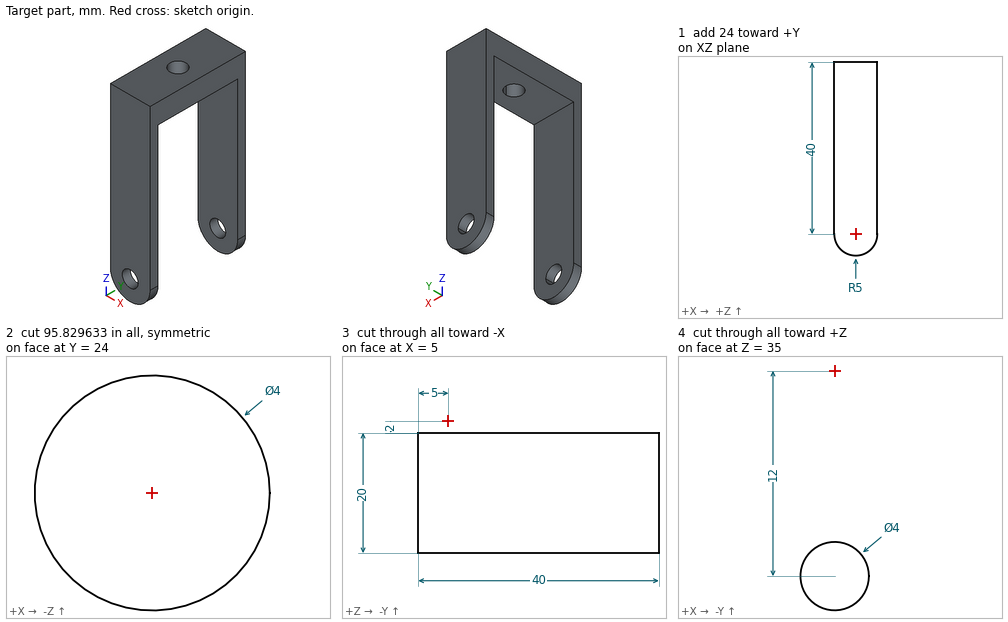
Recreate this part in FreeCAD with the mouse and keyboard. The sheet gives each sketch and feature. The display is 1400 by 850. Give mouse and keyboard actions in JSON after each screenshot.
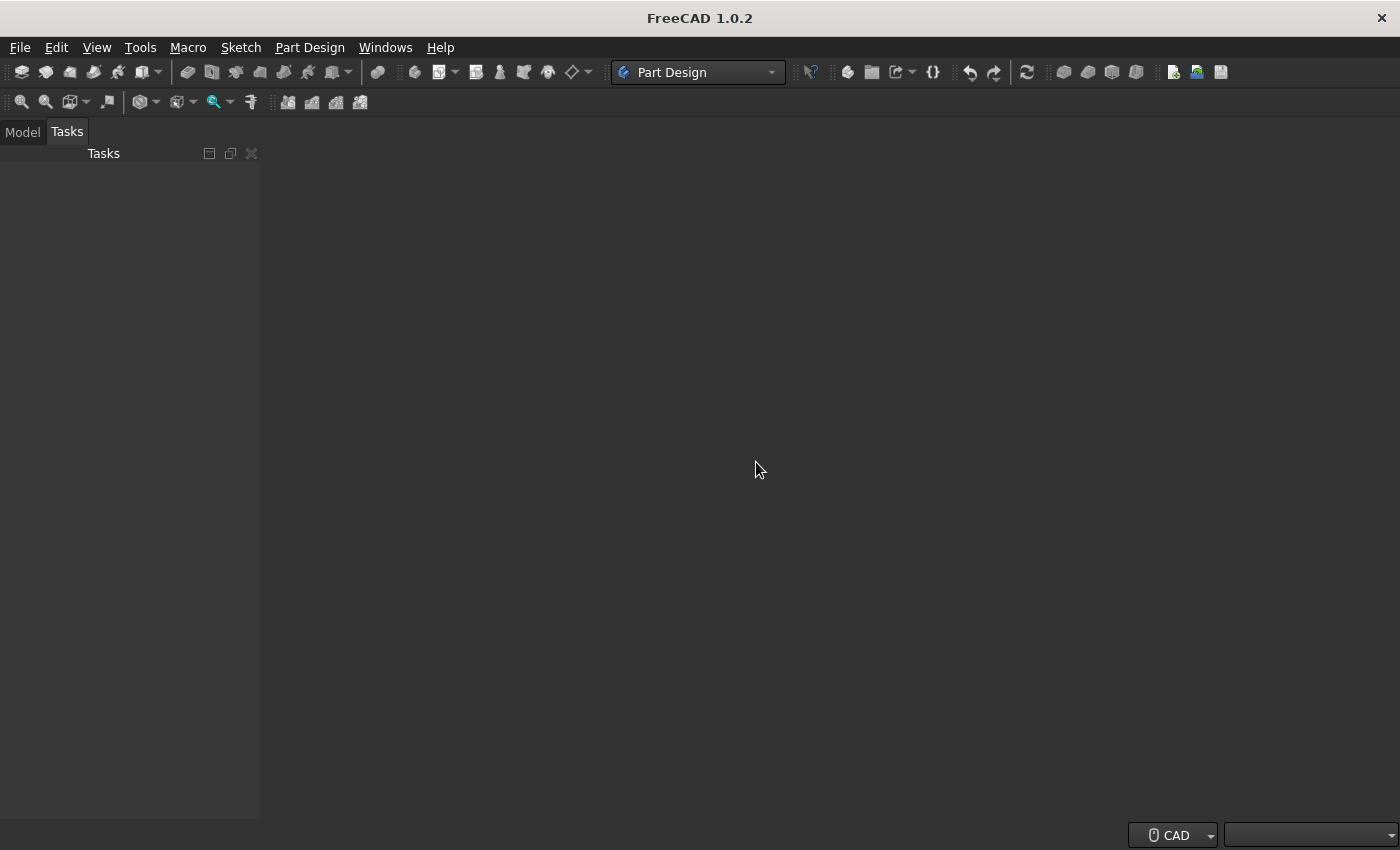
{"action": "left_click", "coordinate": [1174, 72]}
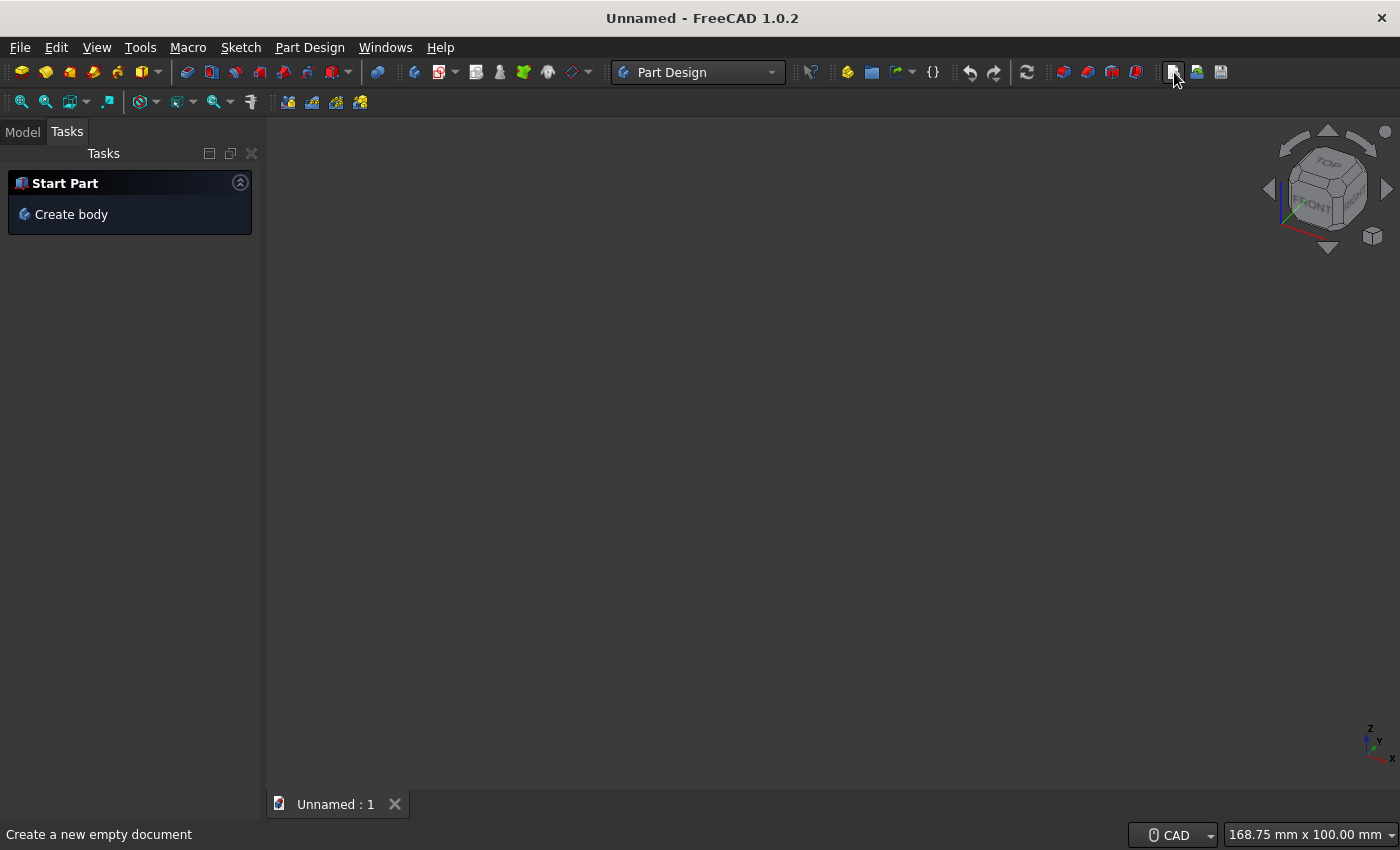
{"action": "left_click", "coordinate": [440, 72]}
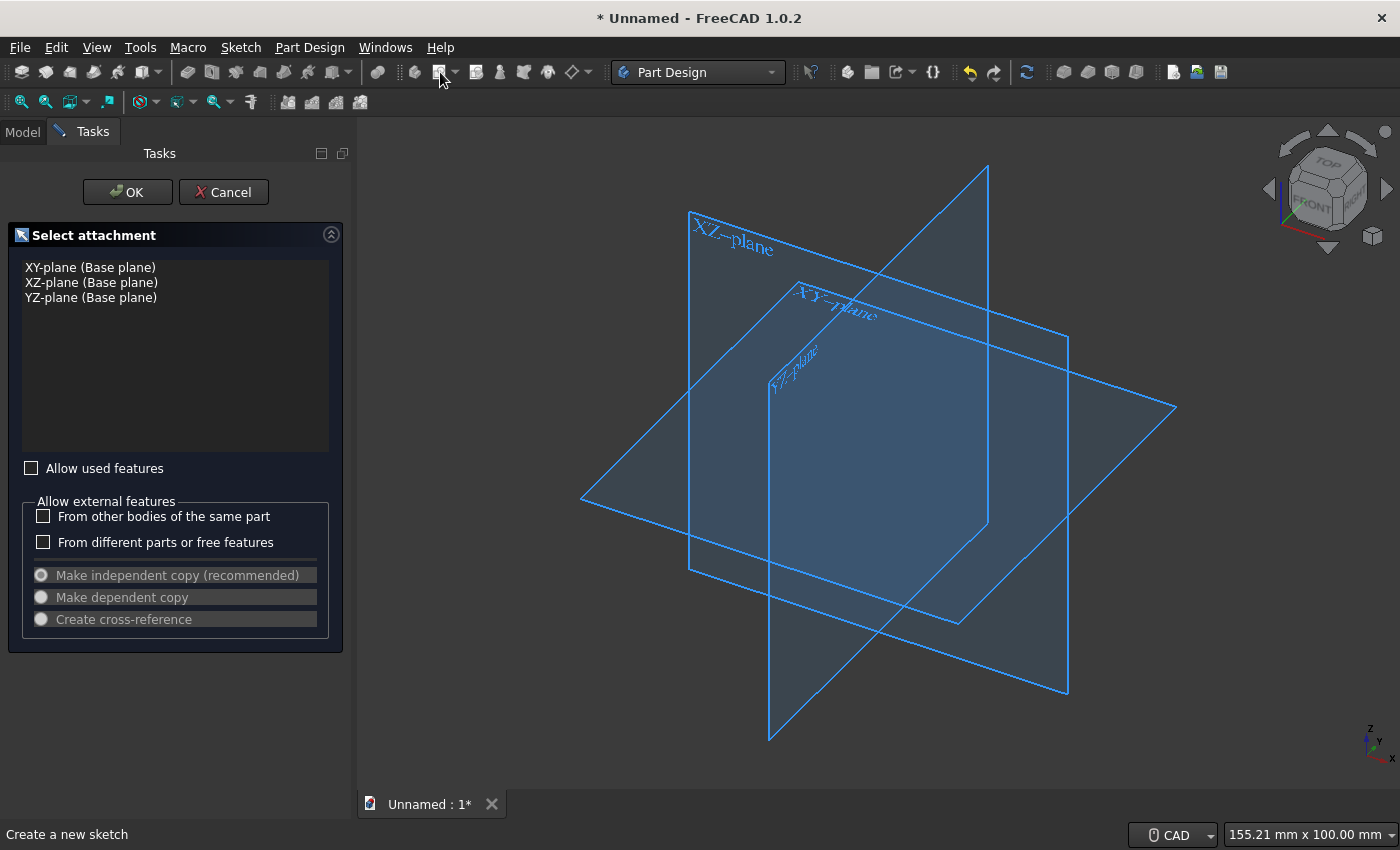
{"action": "left_click", "coordinate": [82, 282]}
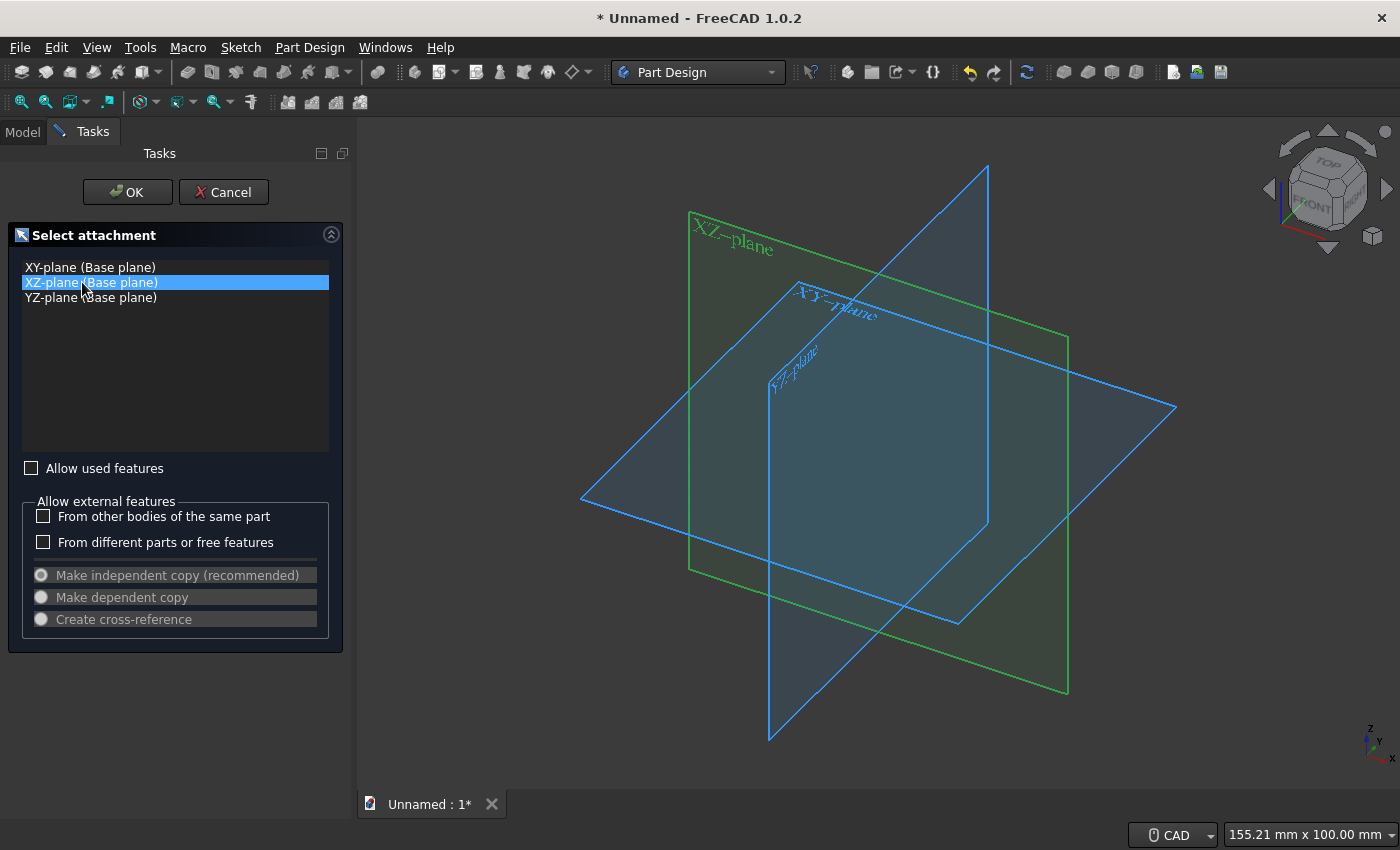
{"action": "left_click", "coordinate": [128, 192]}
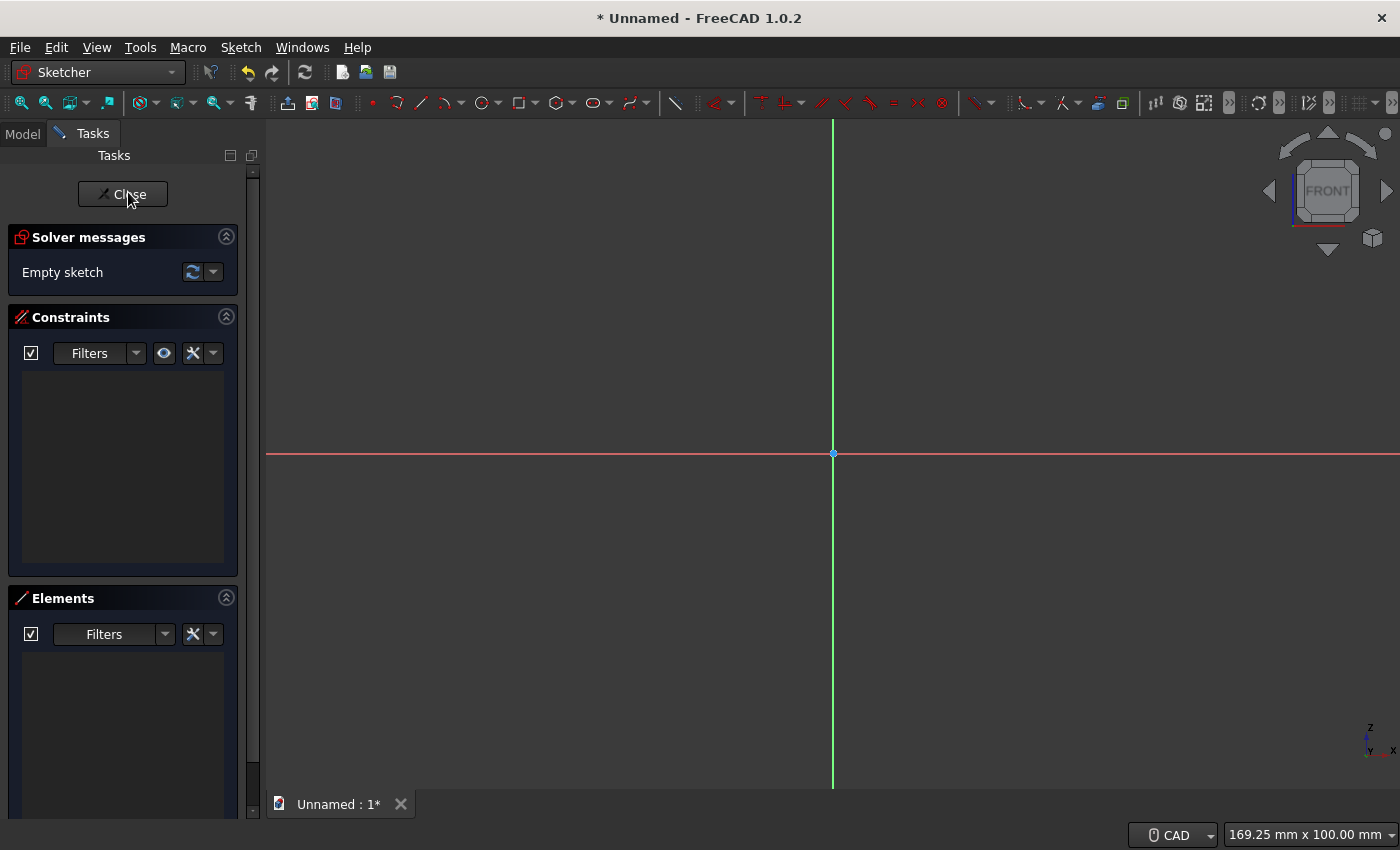
{"action": "scroll", "coordinate": [972, 147], "scroll_direction": "up", "scroll_amount": 2}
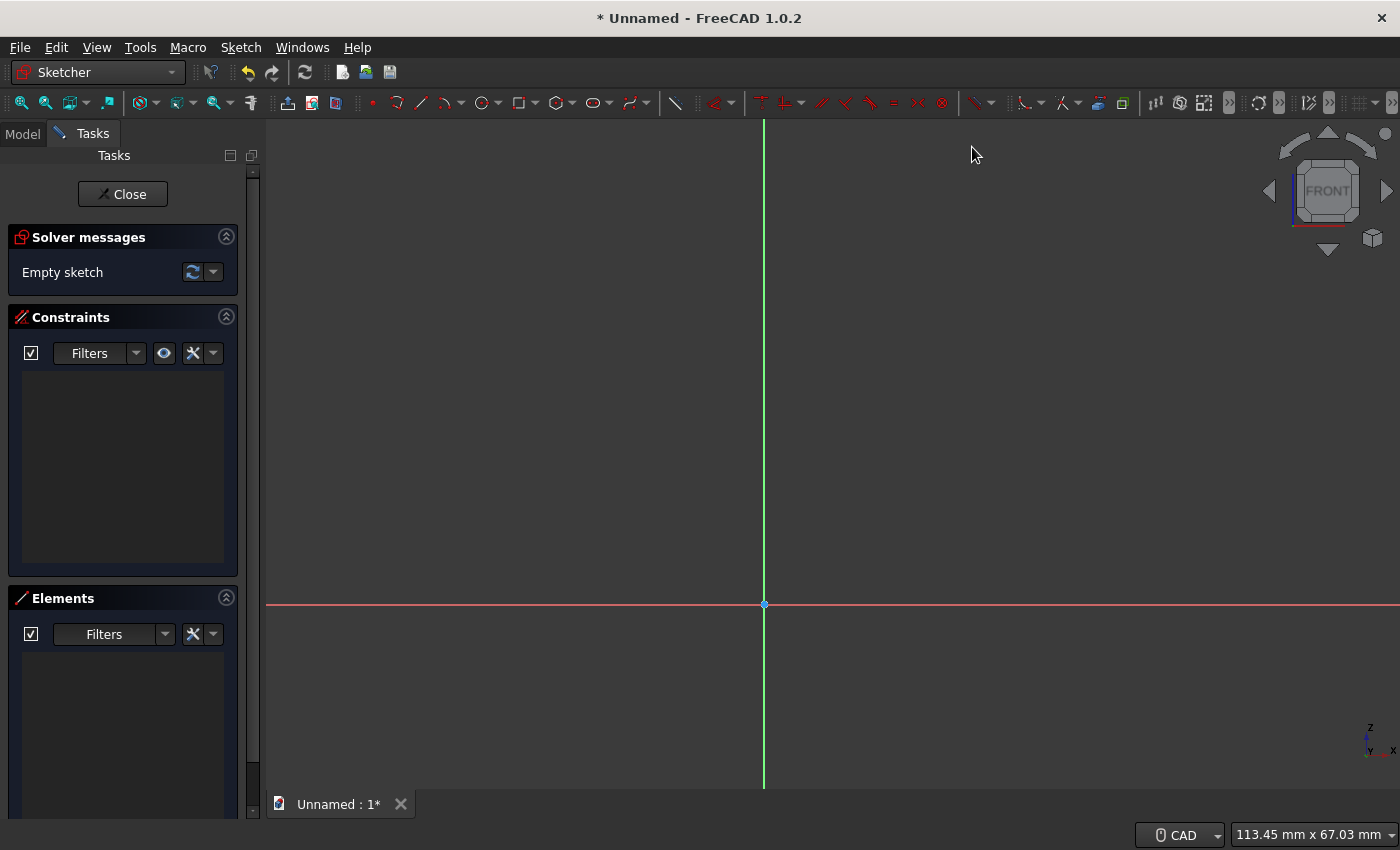
{"action": "key", "text": "g m"}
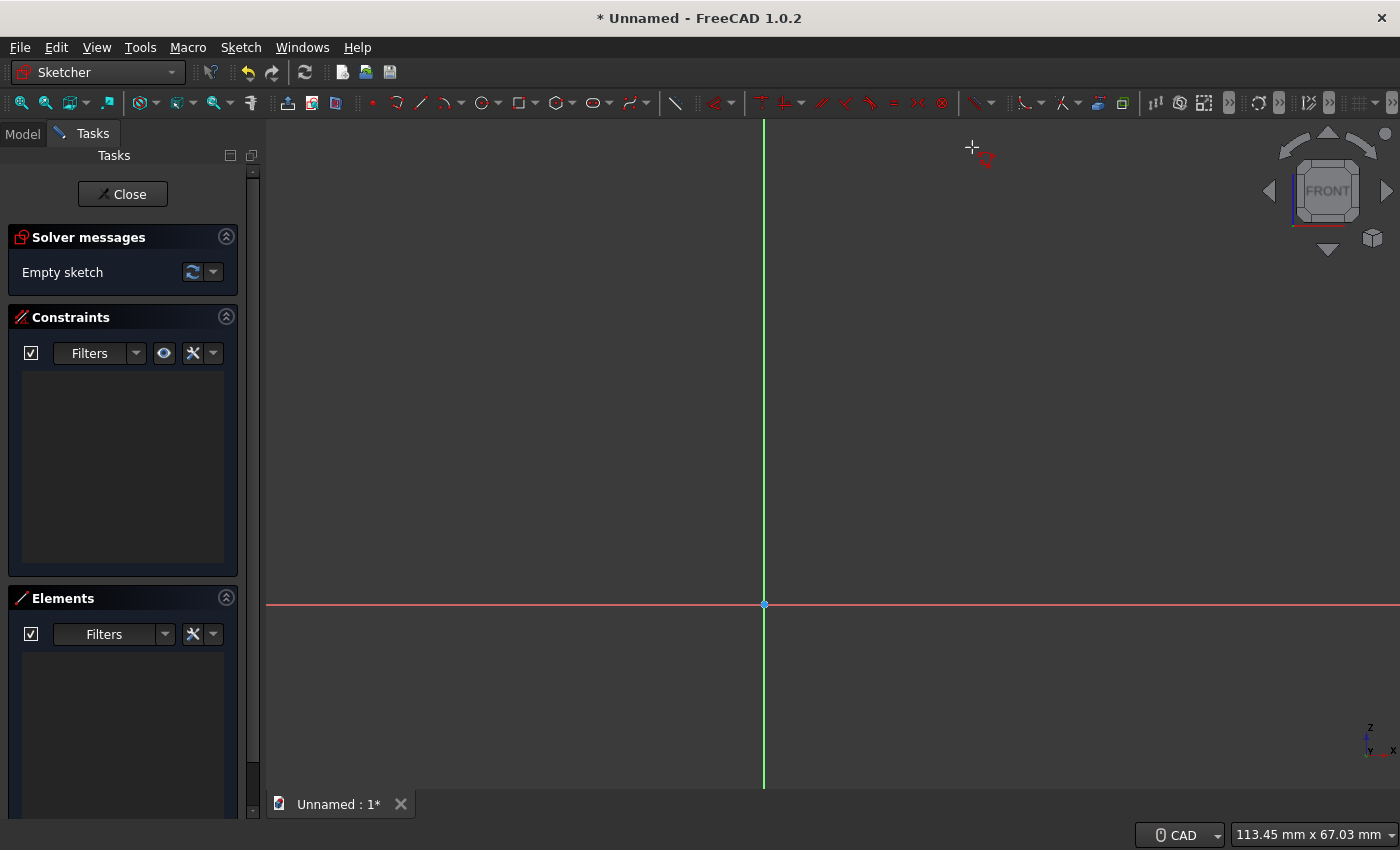
{"action": "left_click", "coordinate": [714, 605]}
{"action": "left_click", "coordinate": [714, 205]}
{"action": "left_click", "coordinate": [814, 205]}
{"action": "left_click", "coordinate": [814, 605]}
{"action": "right_click", "coordinate": [814, 605]}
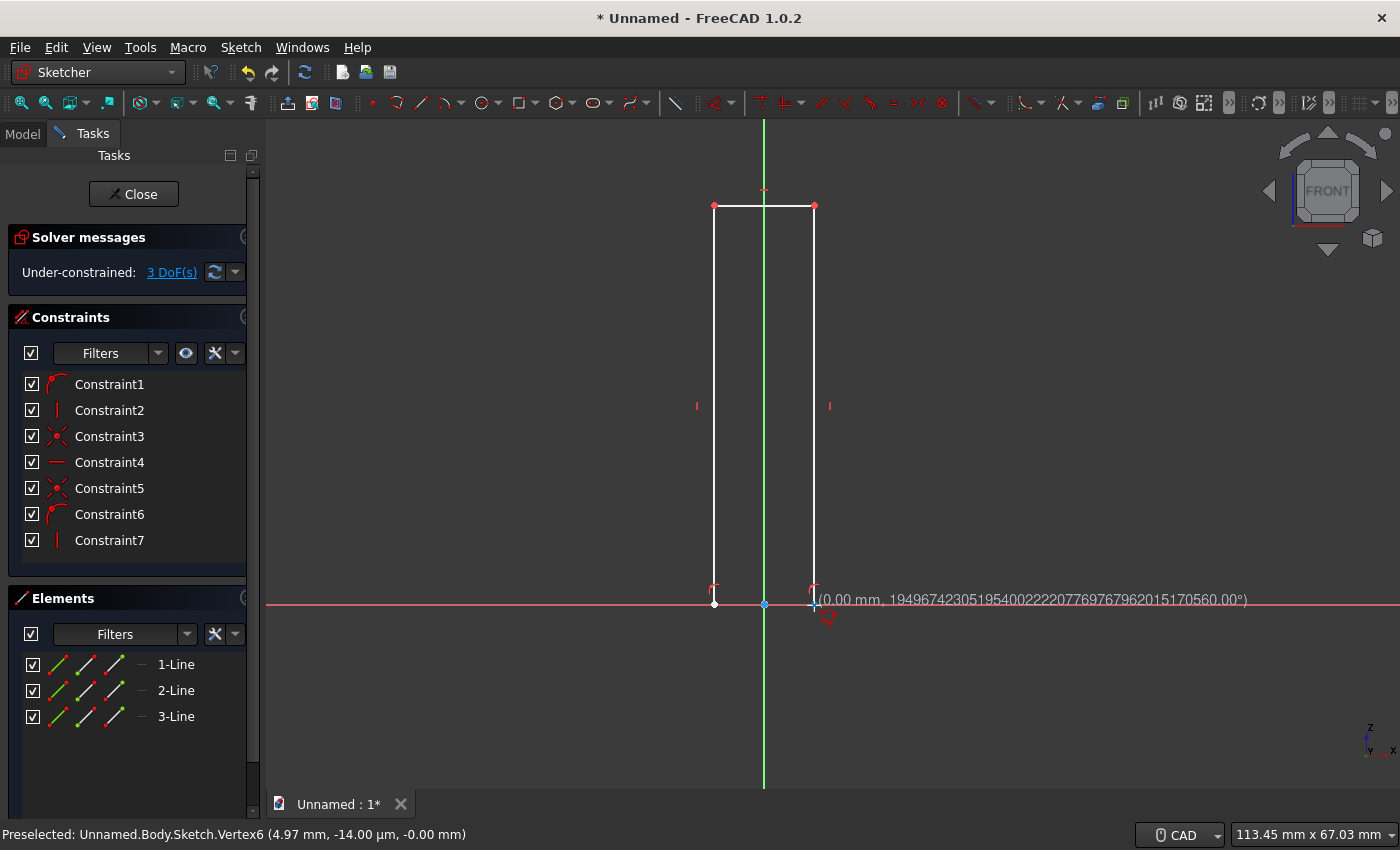
{"action": "key", "text": "g 3 a"}